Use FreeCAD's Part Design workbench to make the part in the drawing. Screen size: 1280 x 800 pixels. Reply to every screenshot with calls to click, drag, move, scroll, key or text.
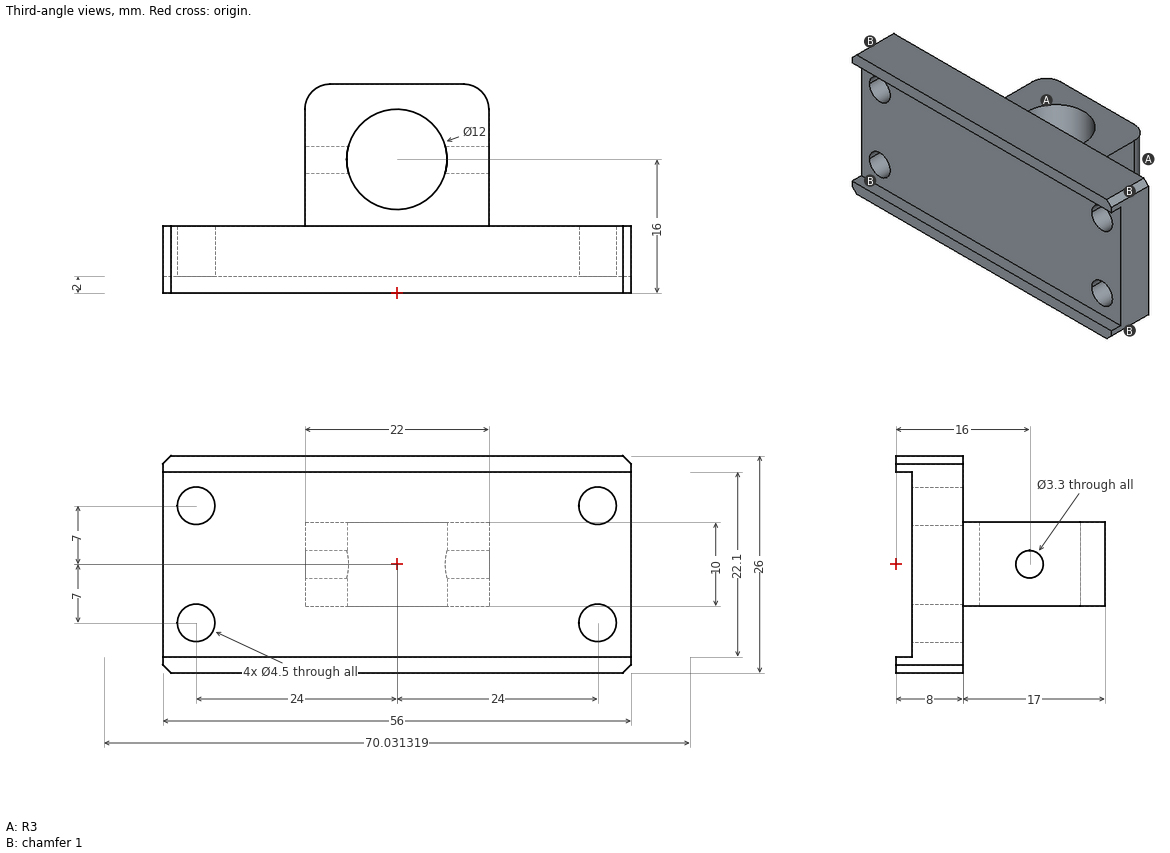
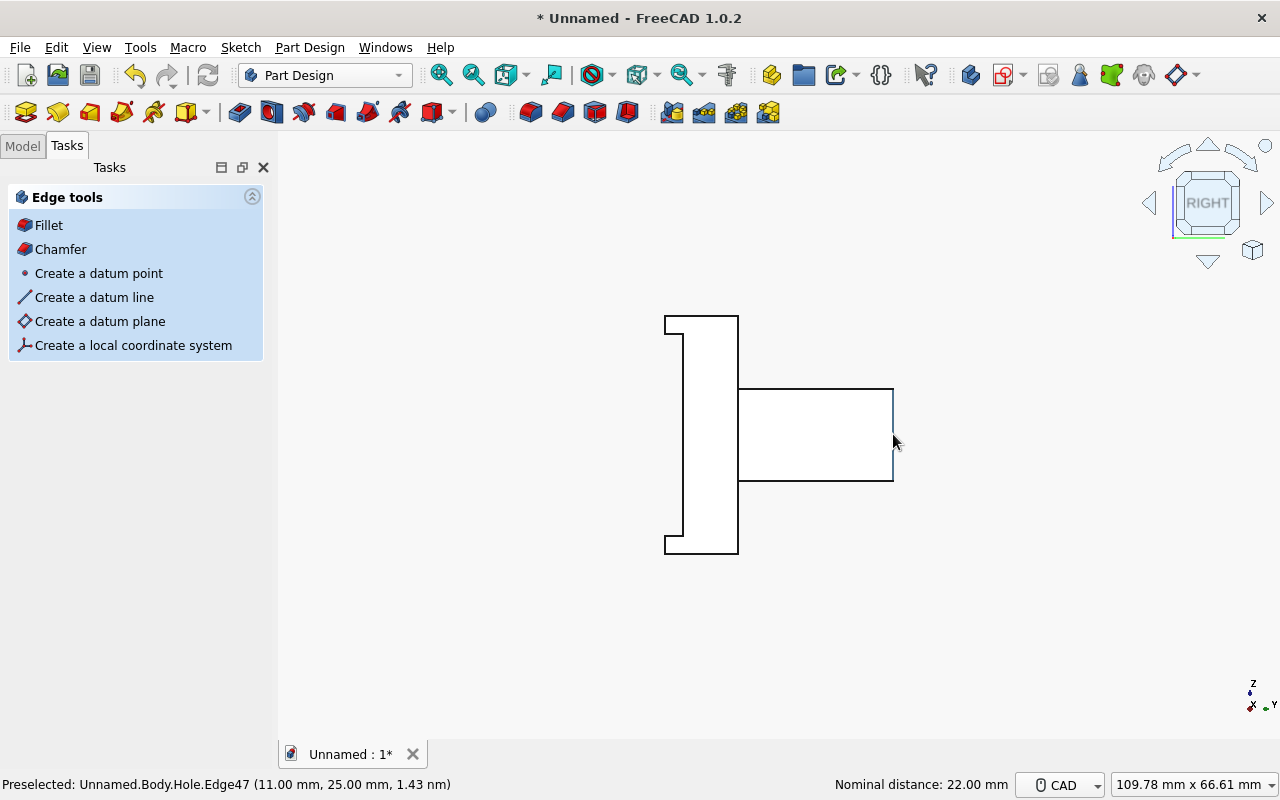
click(532, 112)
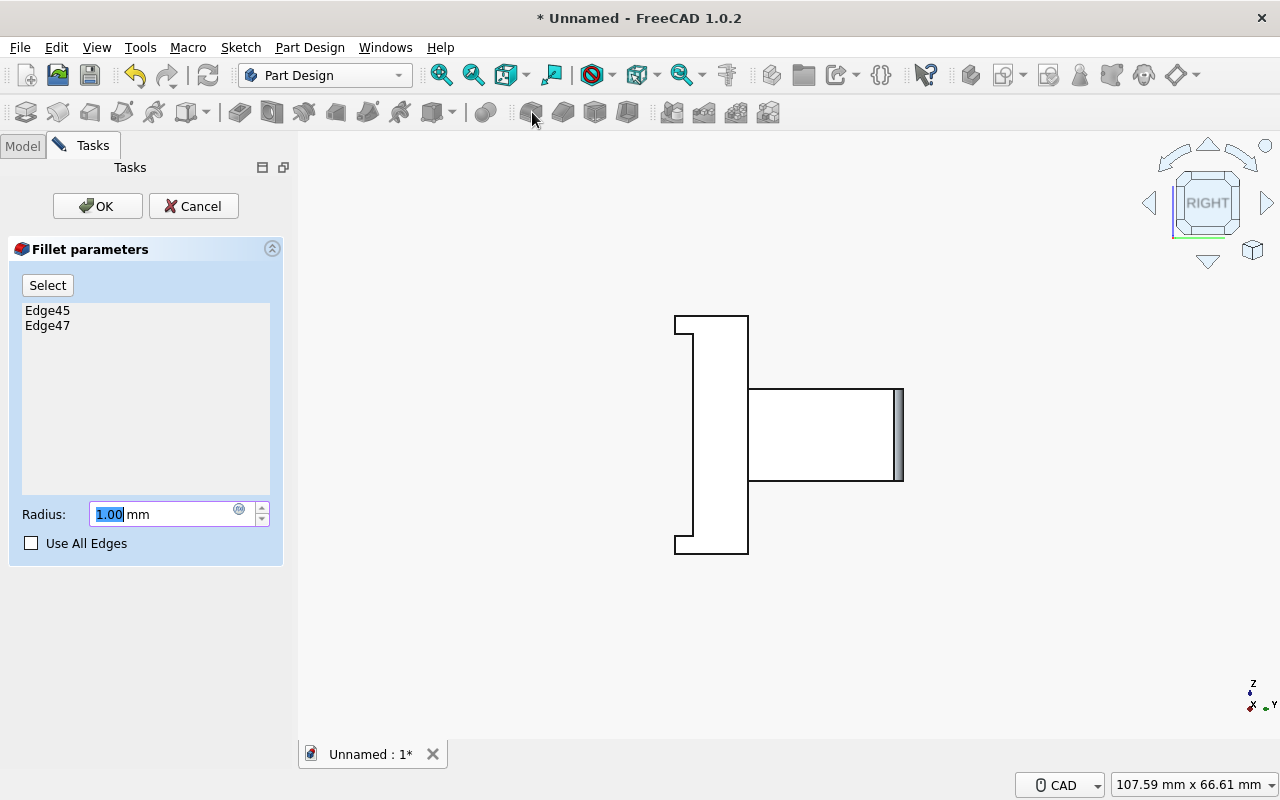
text(3)
key(Tab)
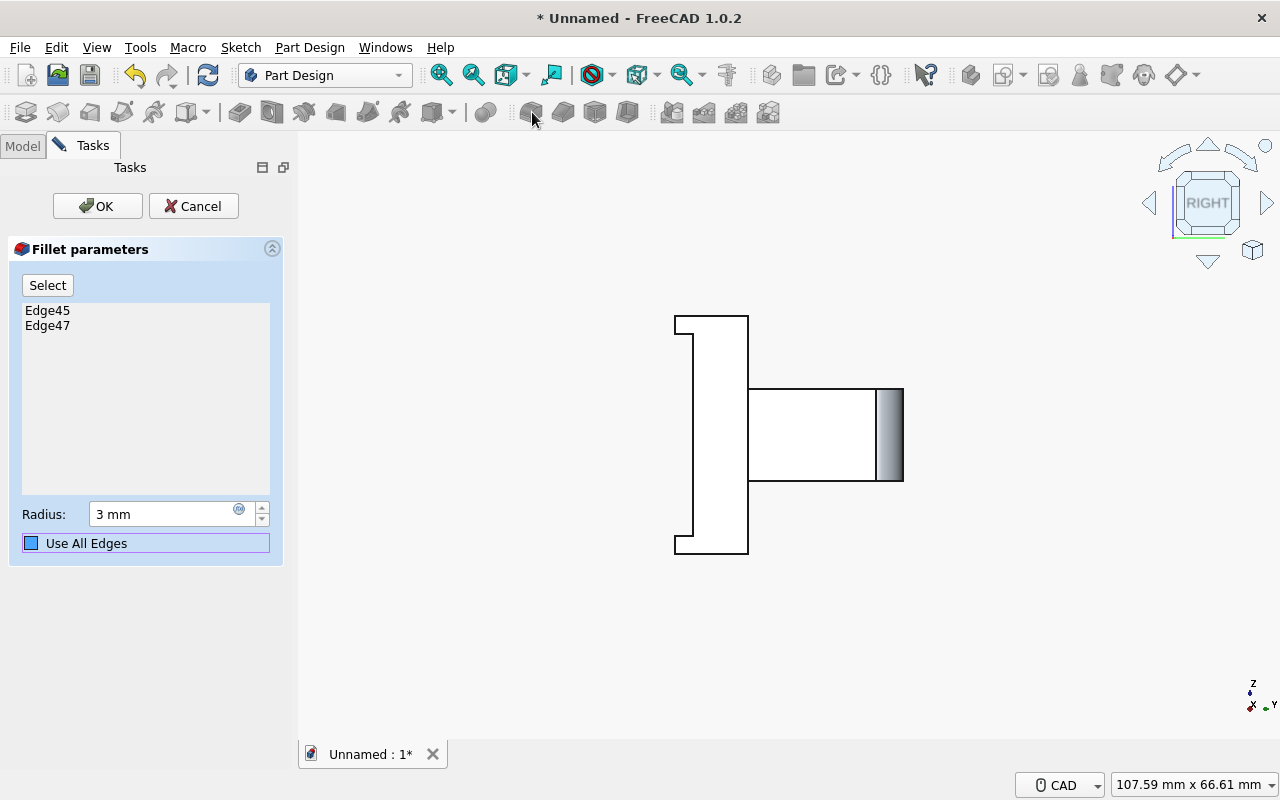
click(98, 206)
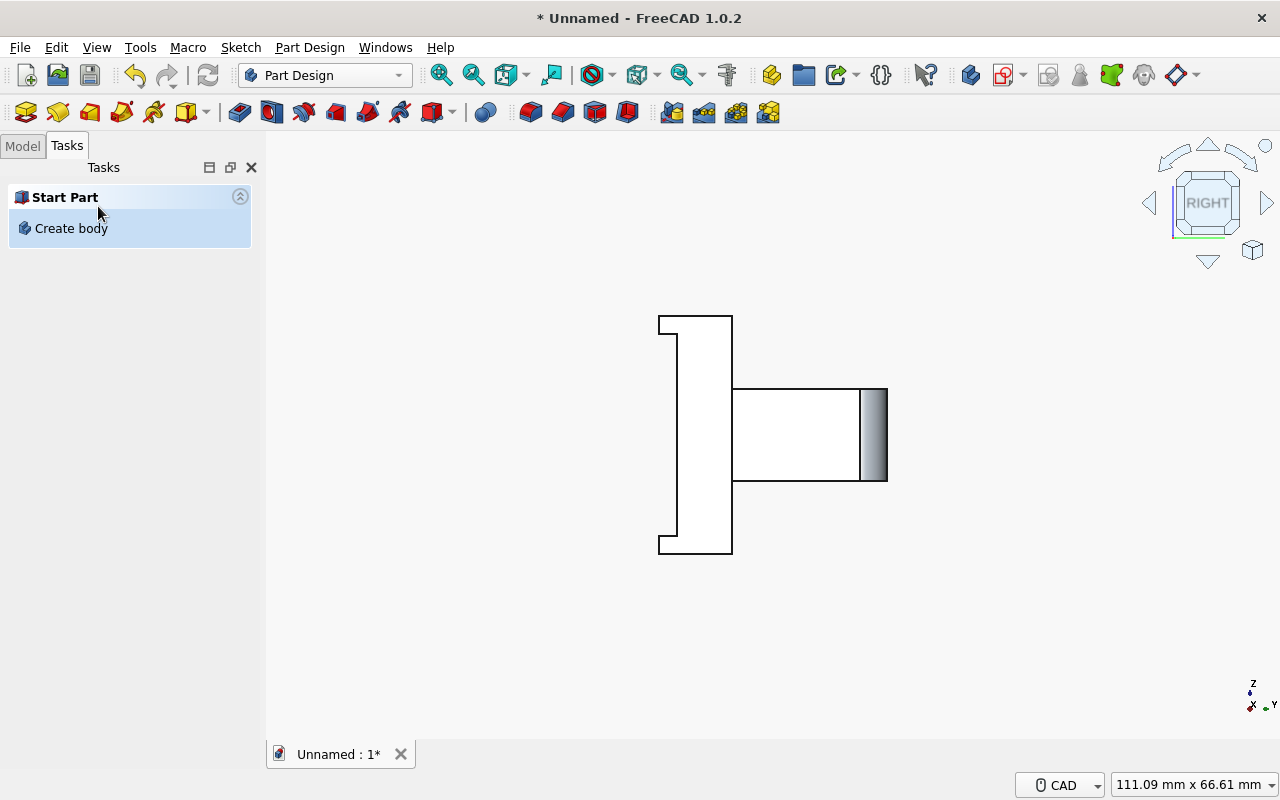
click(442, 76)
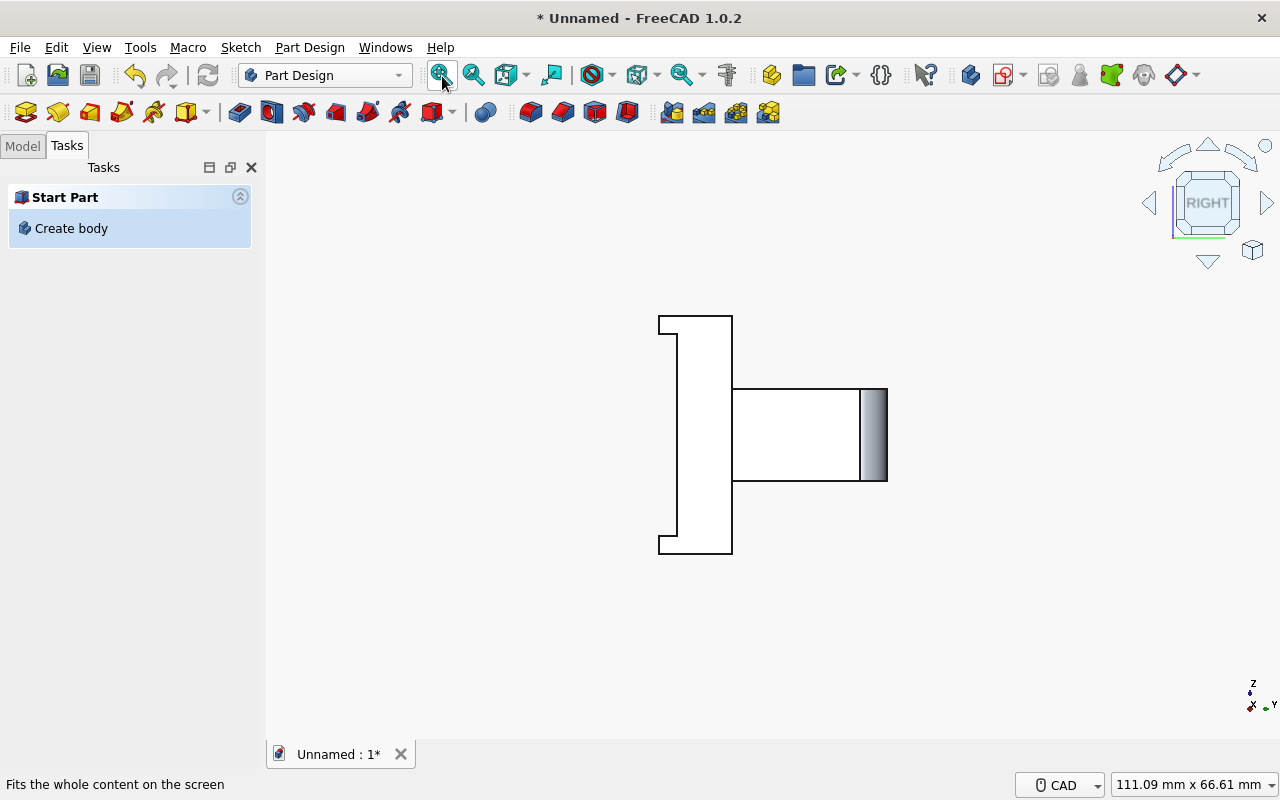
click(796, 434)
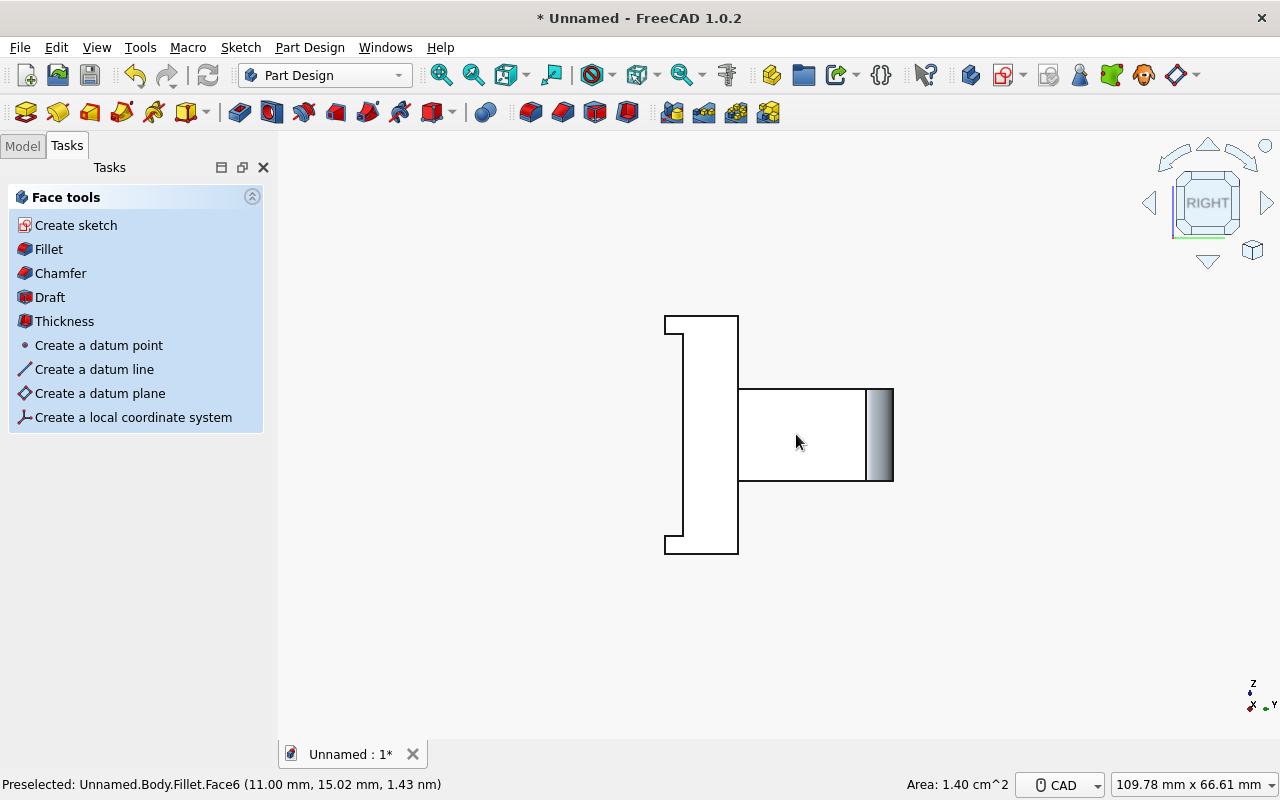
click(1004, 76)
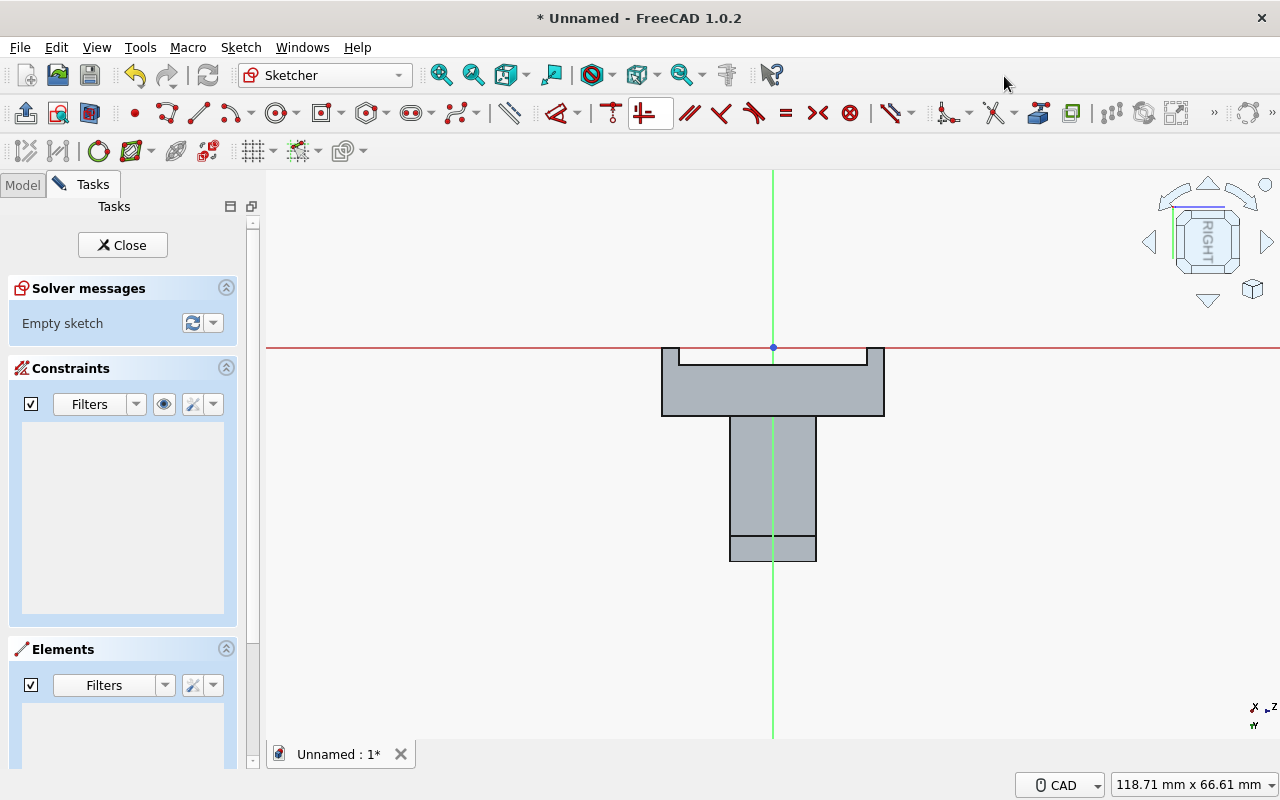
scroll(778, 487, up, 13)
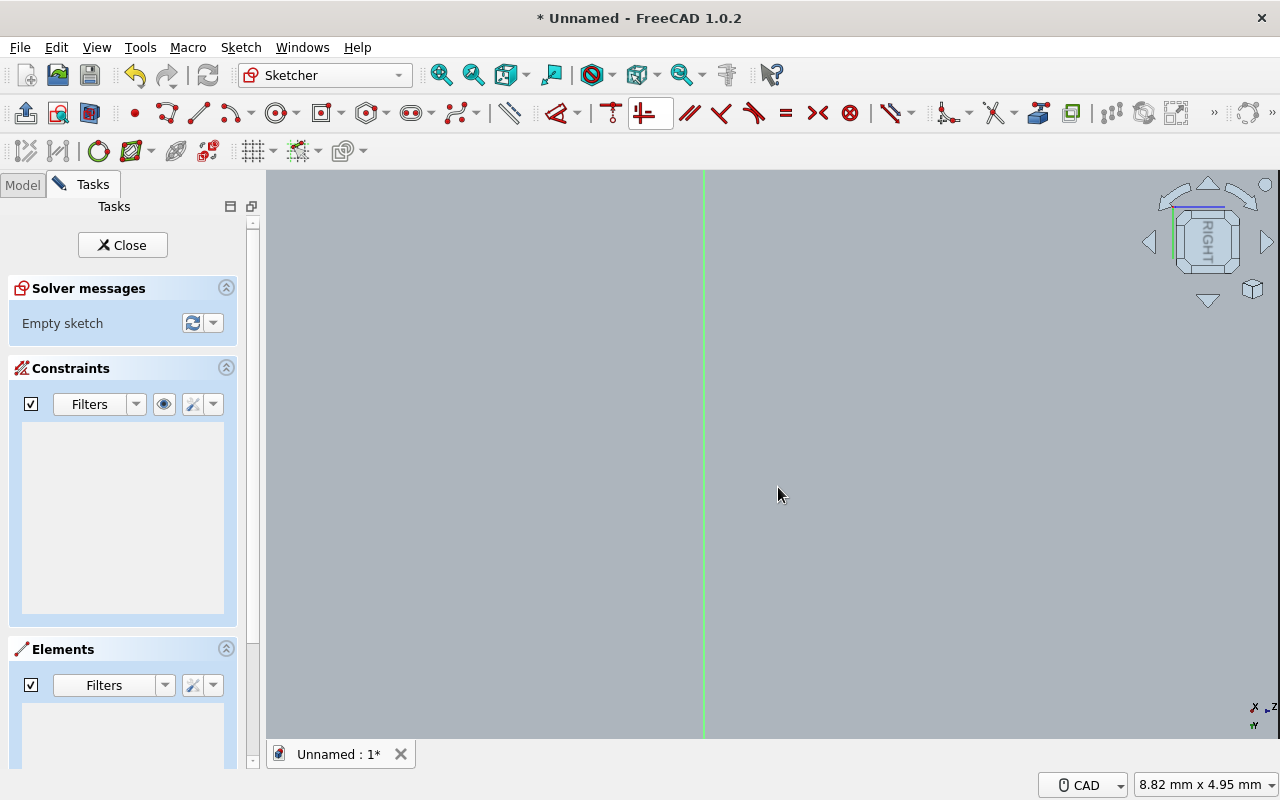
click(276, 114)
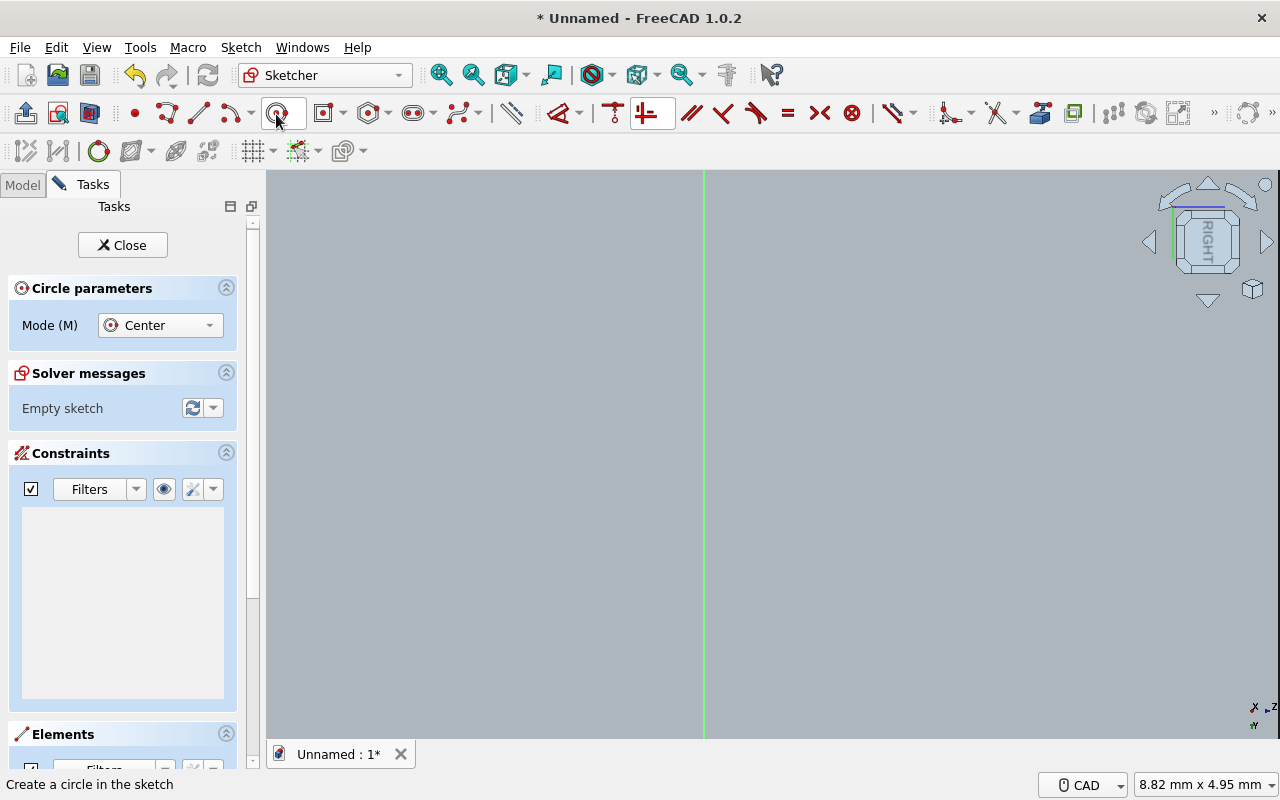
click(704, 445)
move(839, 311)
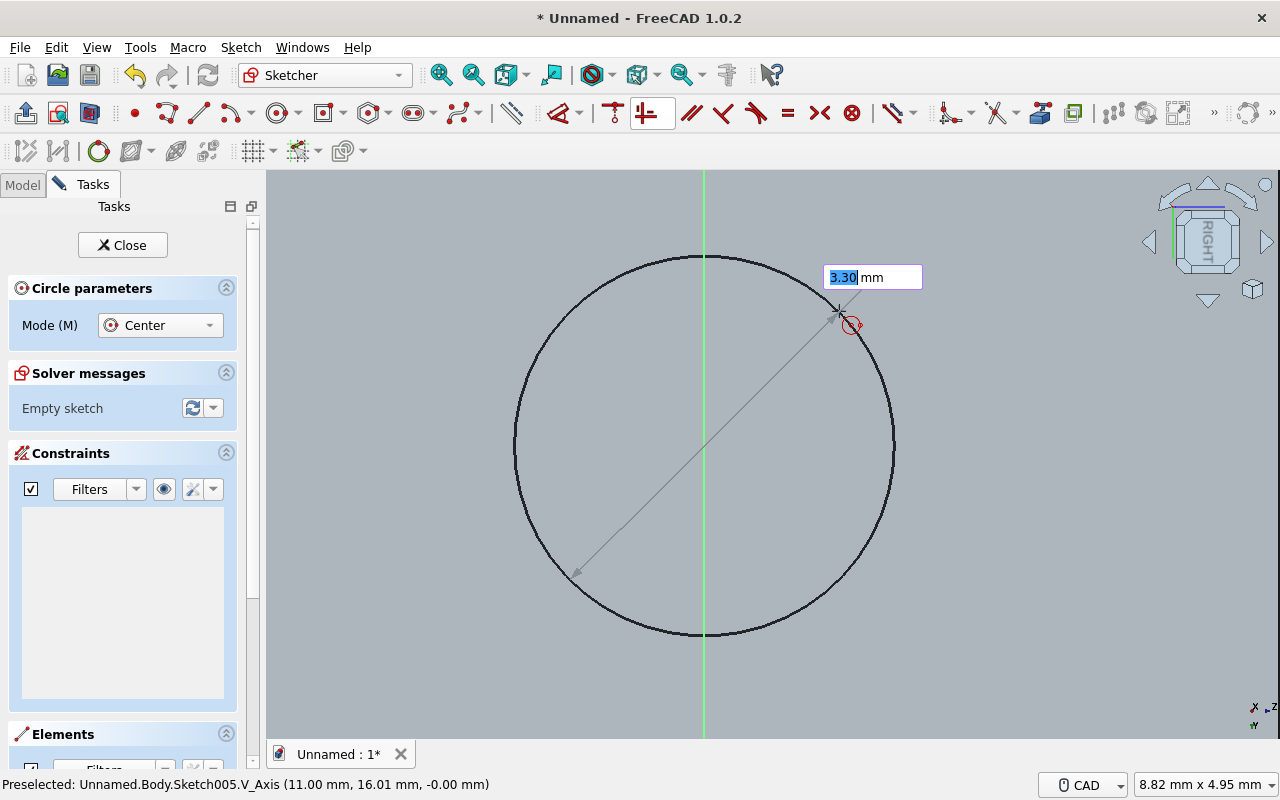
text(3.3)
key(Return)
key(Escape)